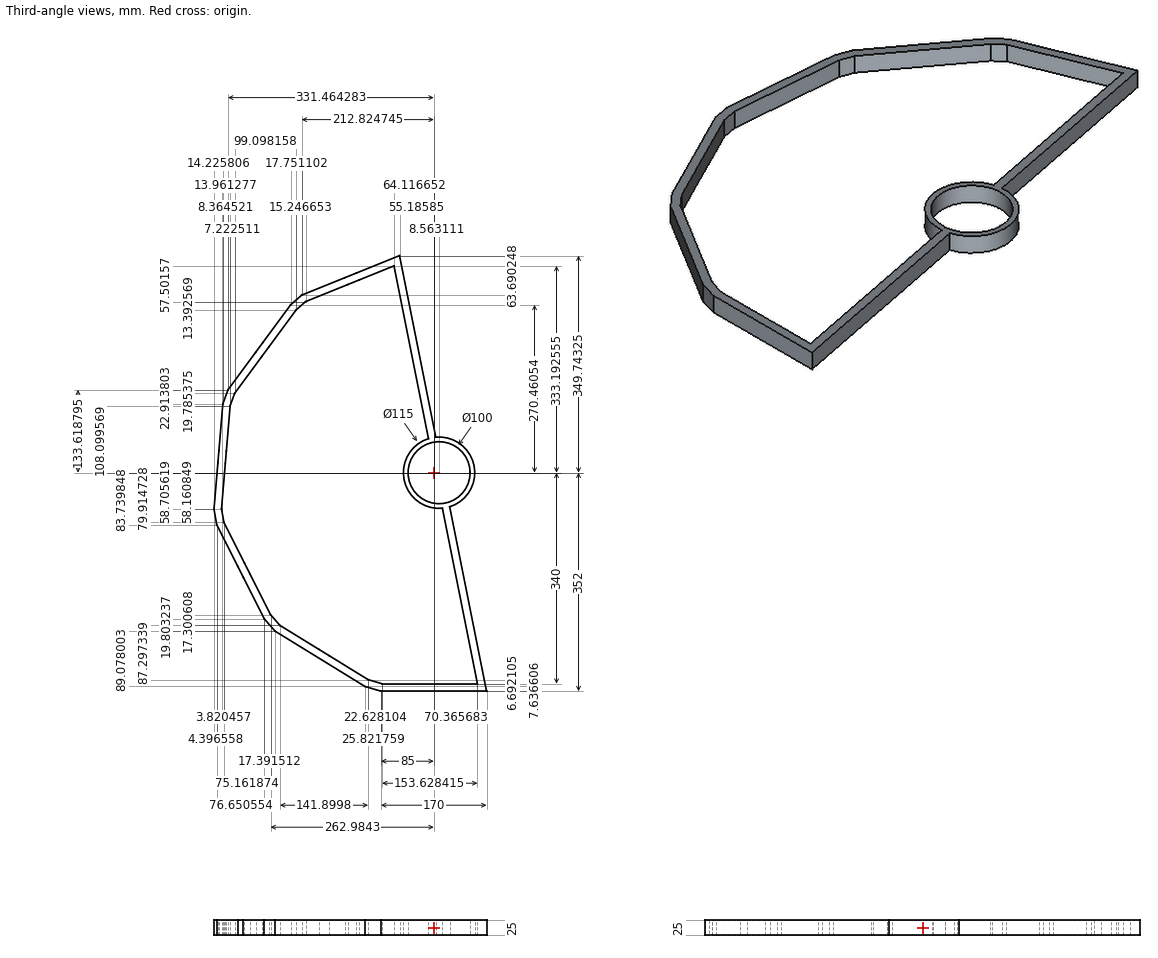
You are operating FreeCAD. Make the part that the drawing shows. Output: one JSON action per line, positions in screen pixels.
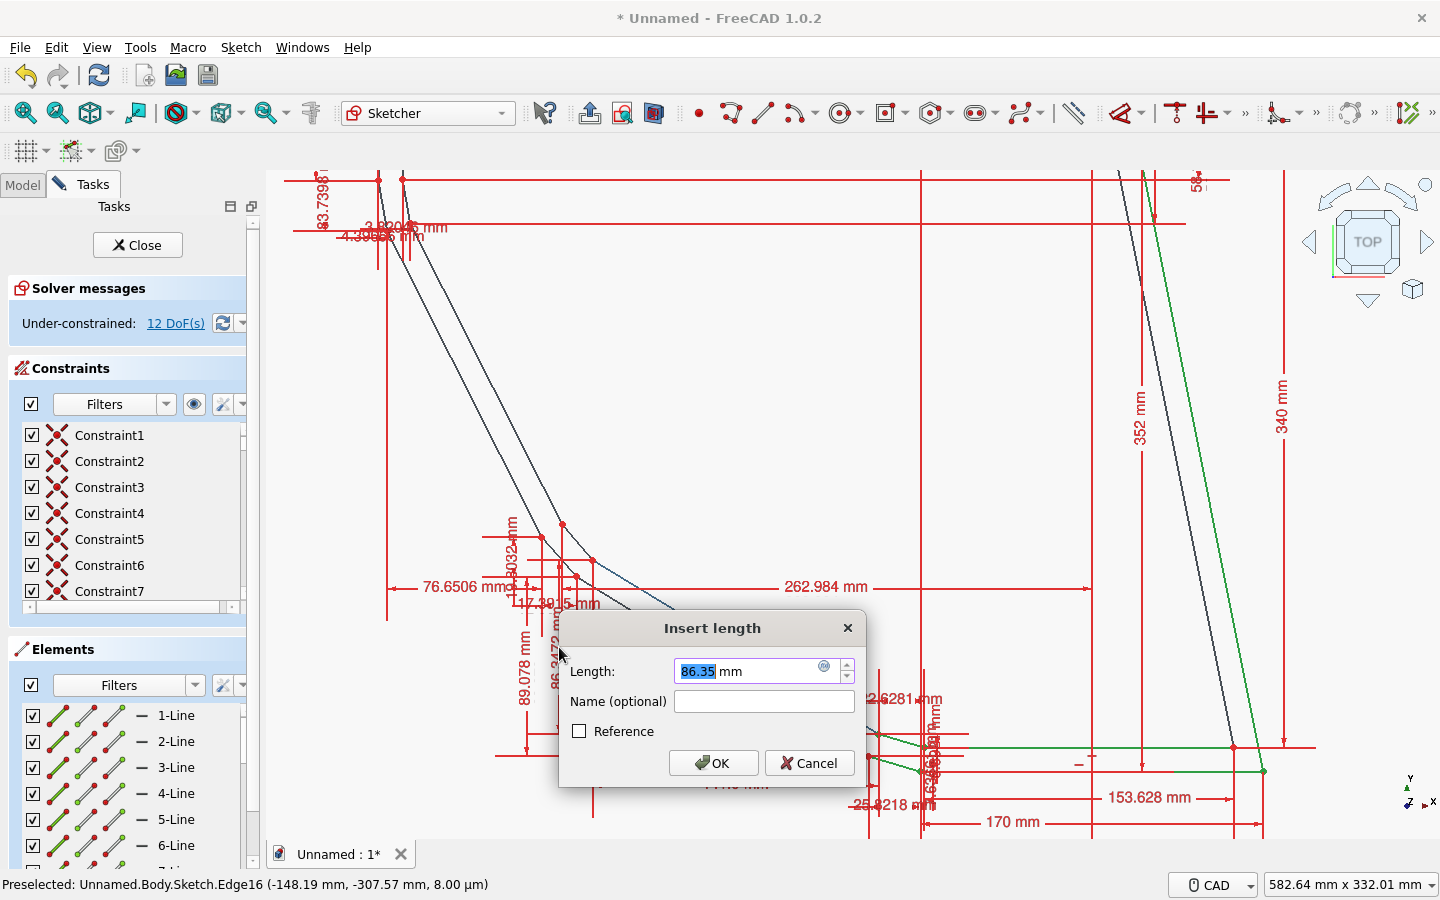
{"action": "type", "text": "87.297339"}
{"action": "key", "text": "Return"}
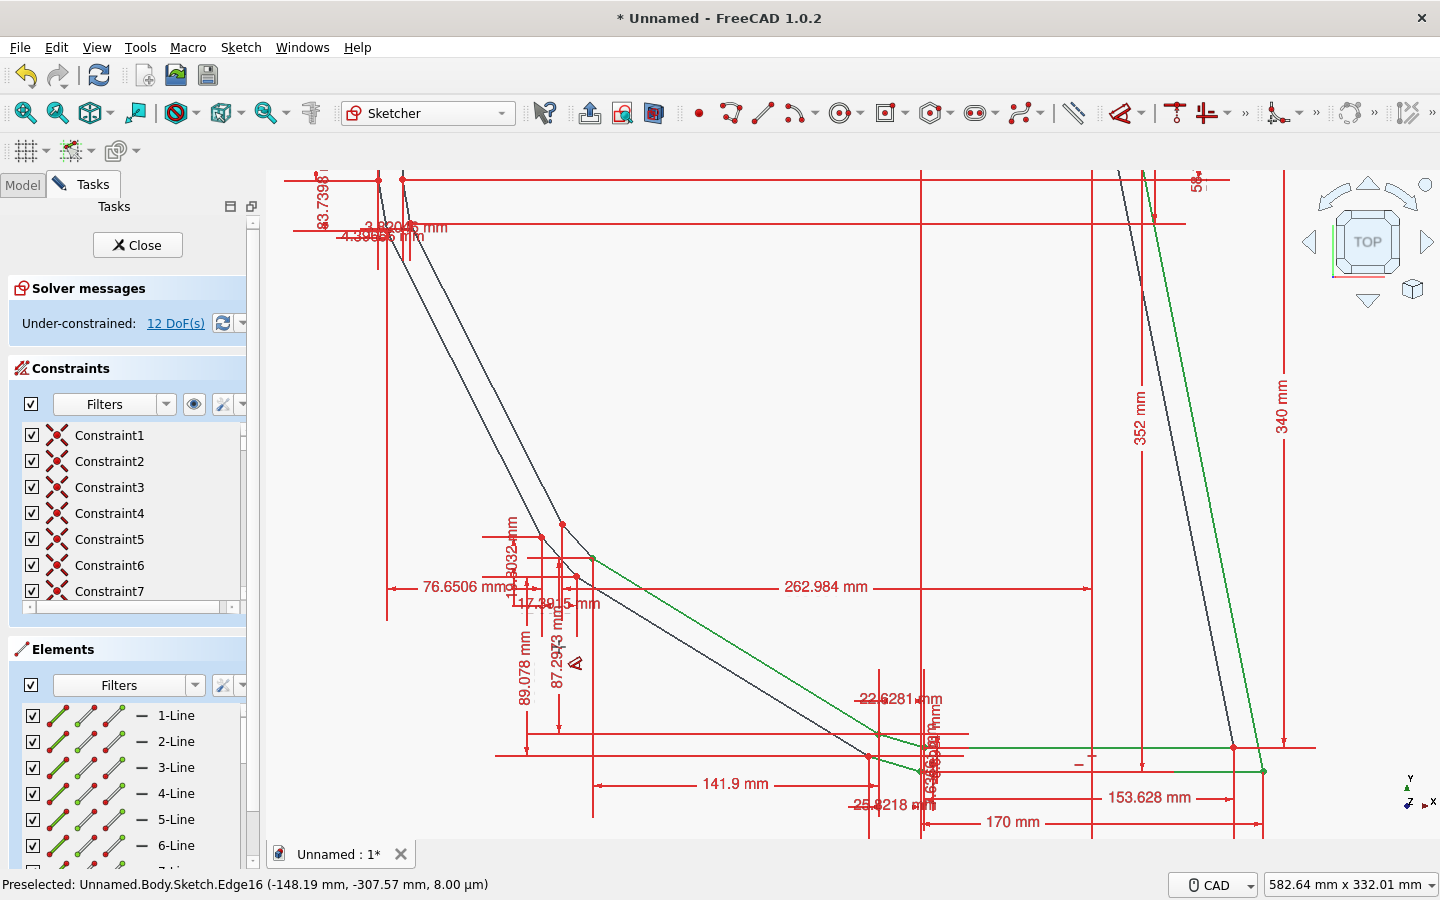
{"action": "left_click", "coordinate": [584, 548]}
{"action": "left_click", "coordinate": [627, 541]}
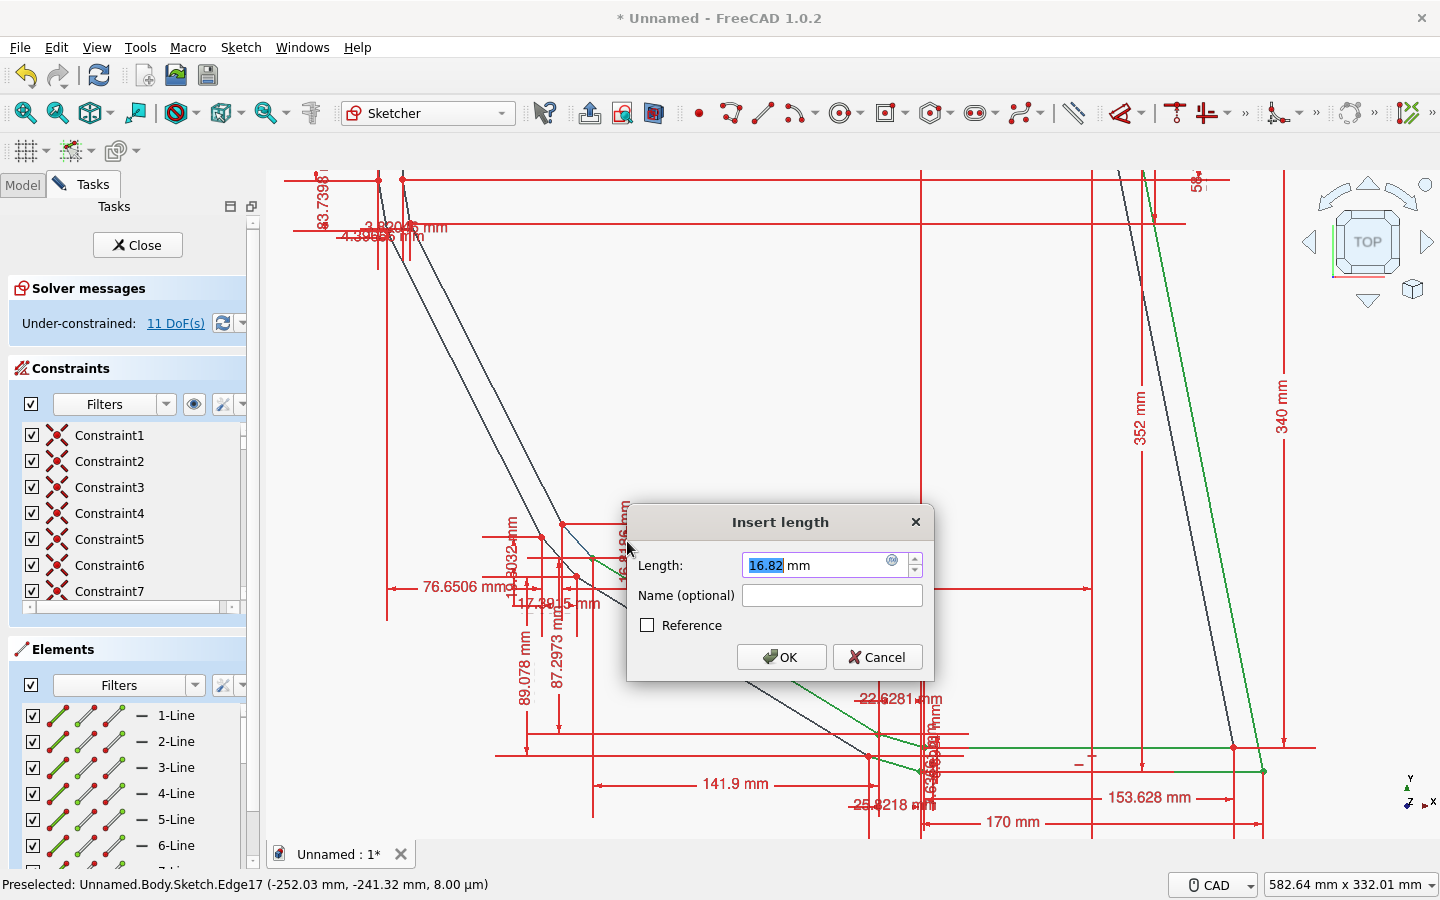
{"action": "type", "text": "17.300608"}
{"action": "key", "text": "Return"}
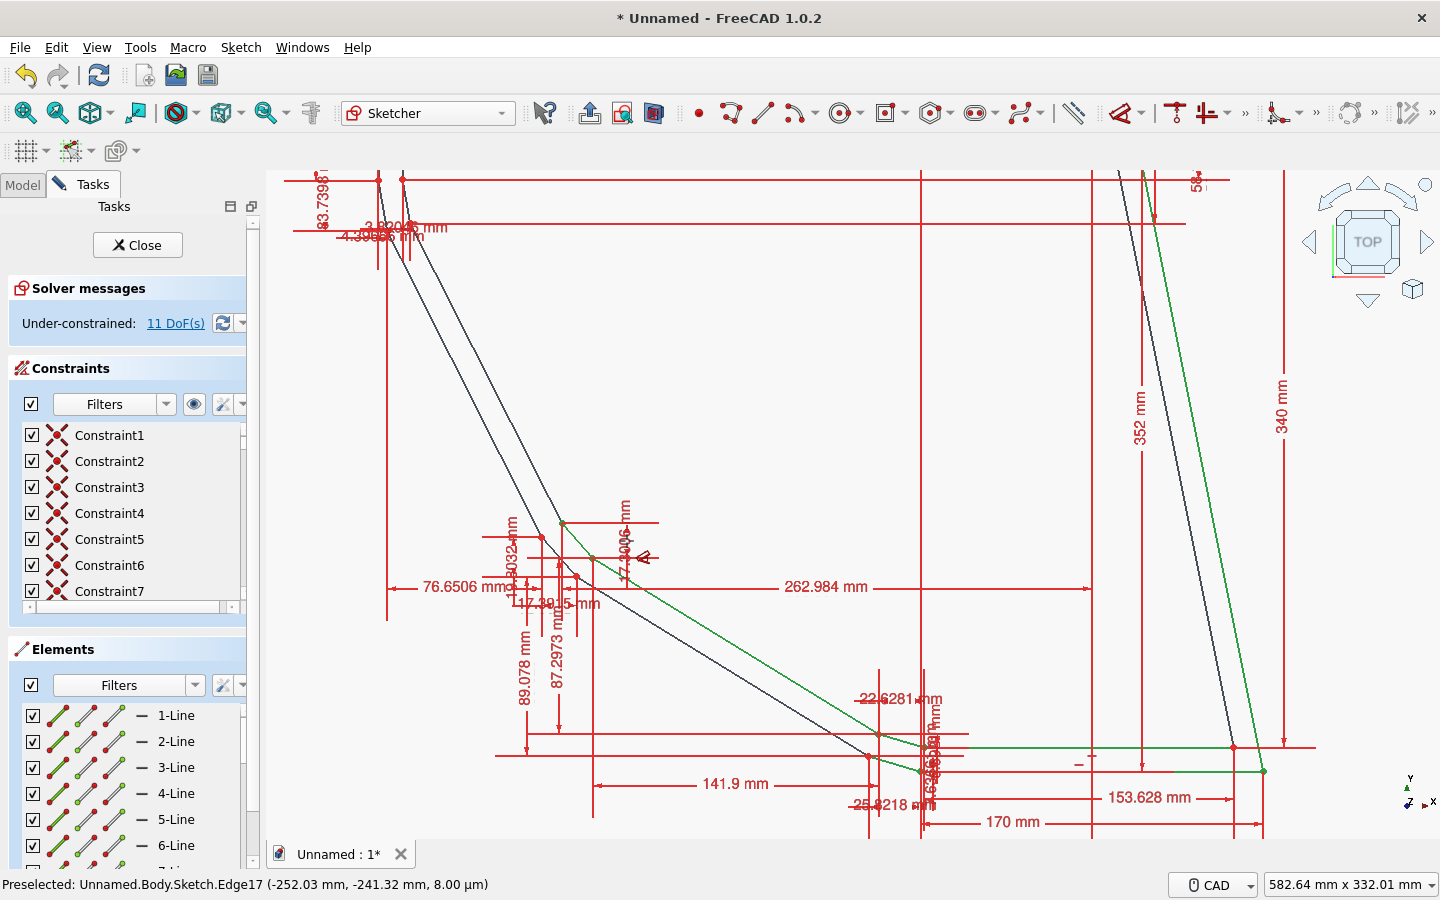
{"action": "left_click", "coordinate": [517, 433]}
{"action": "left_click", "coordinate": [433, 557]}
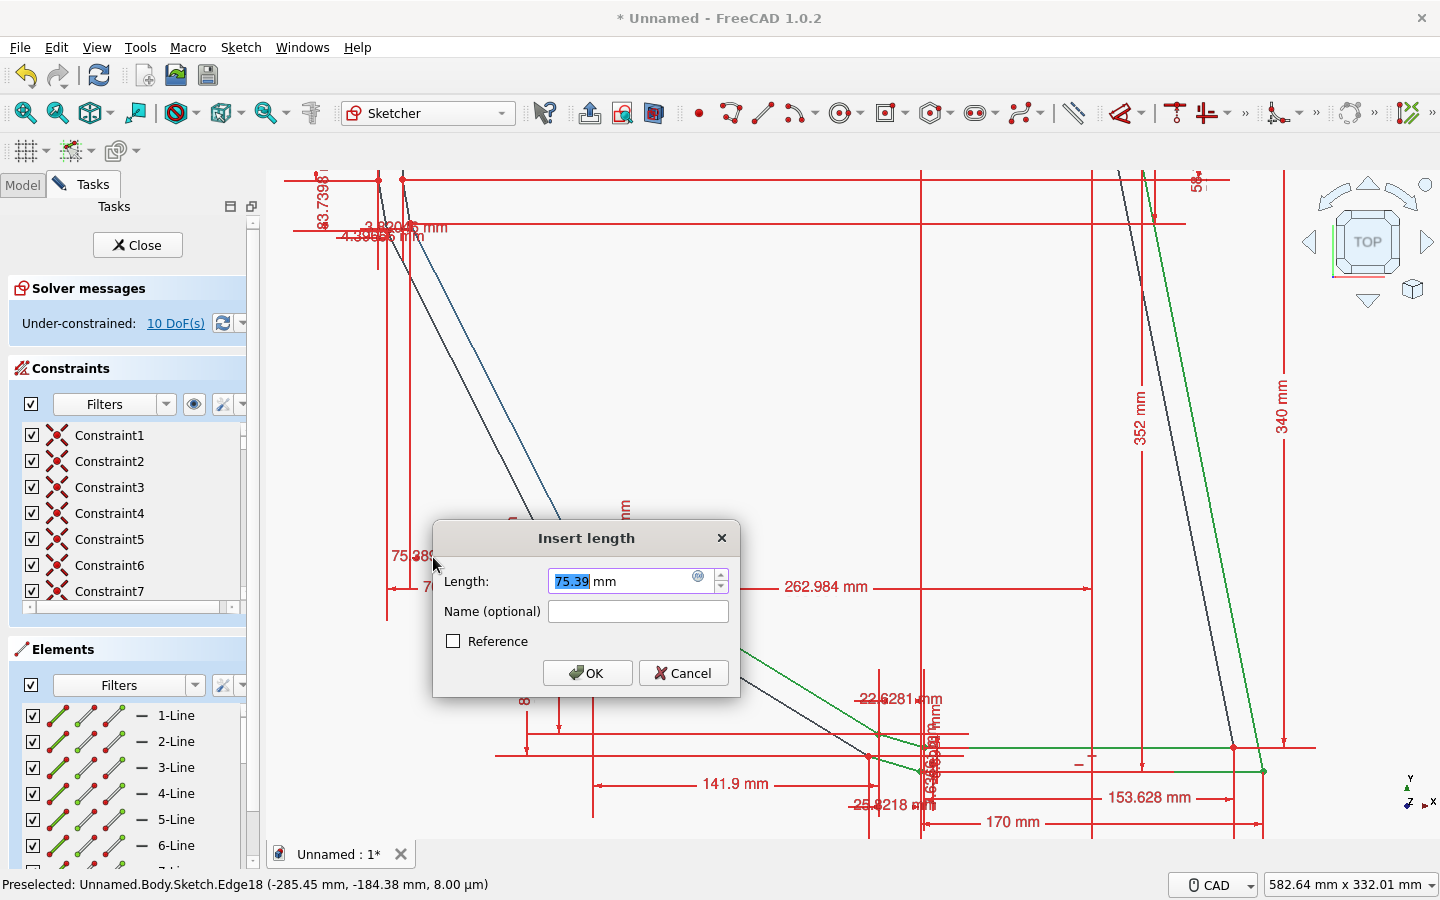
{"action": "type", "text": "75.161874"}
{"action": "key", "text": "Return"}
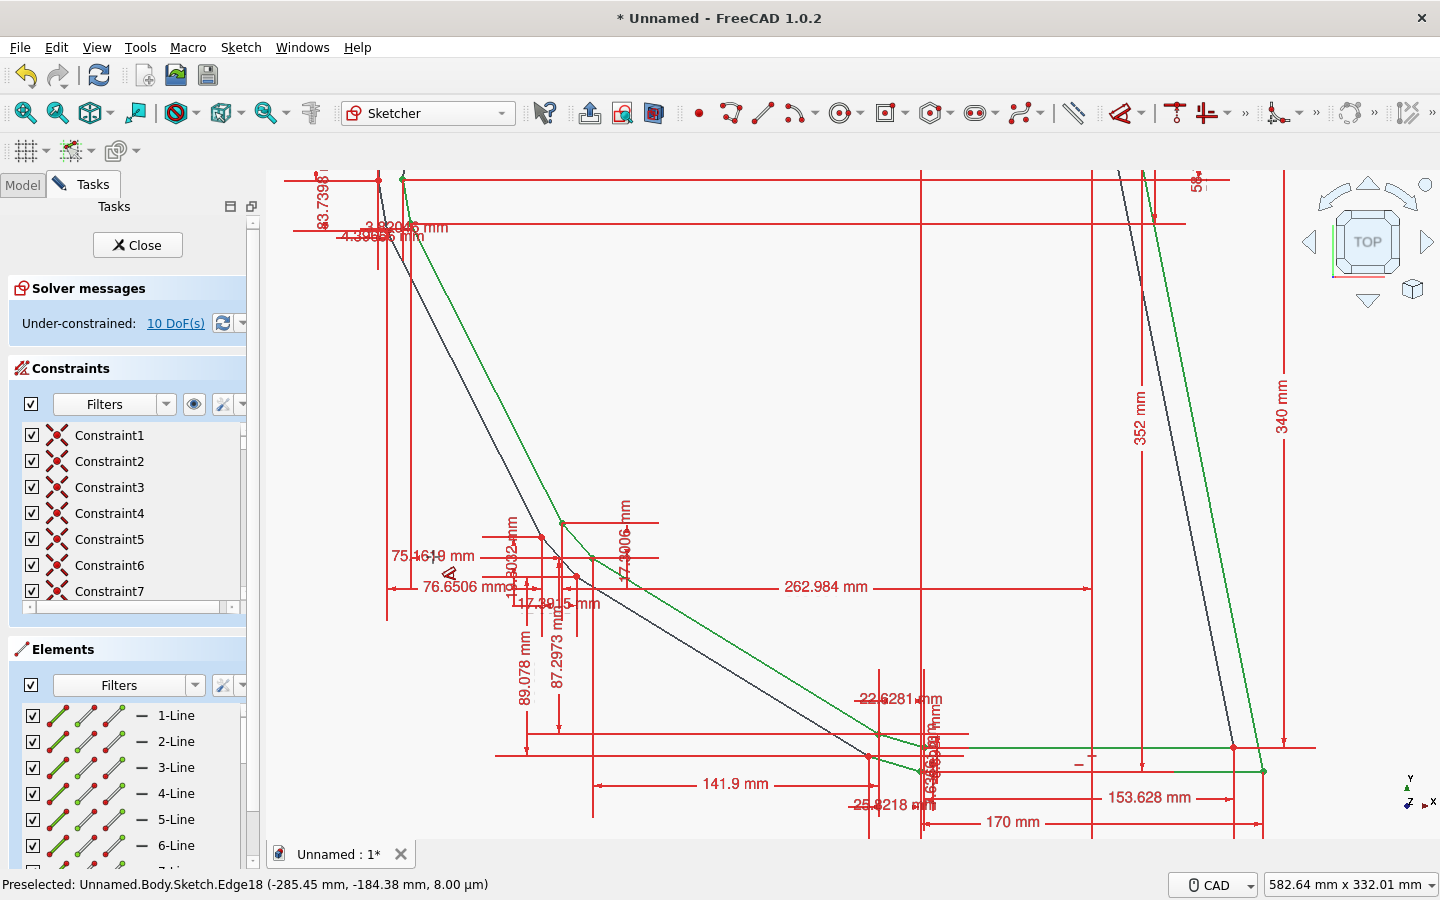
{"action": "scroll", "coordinate": [769, 694], "scroll_direction": "down", "scroll_amount": 6}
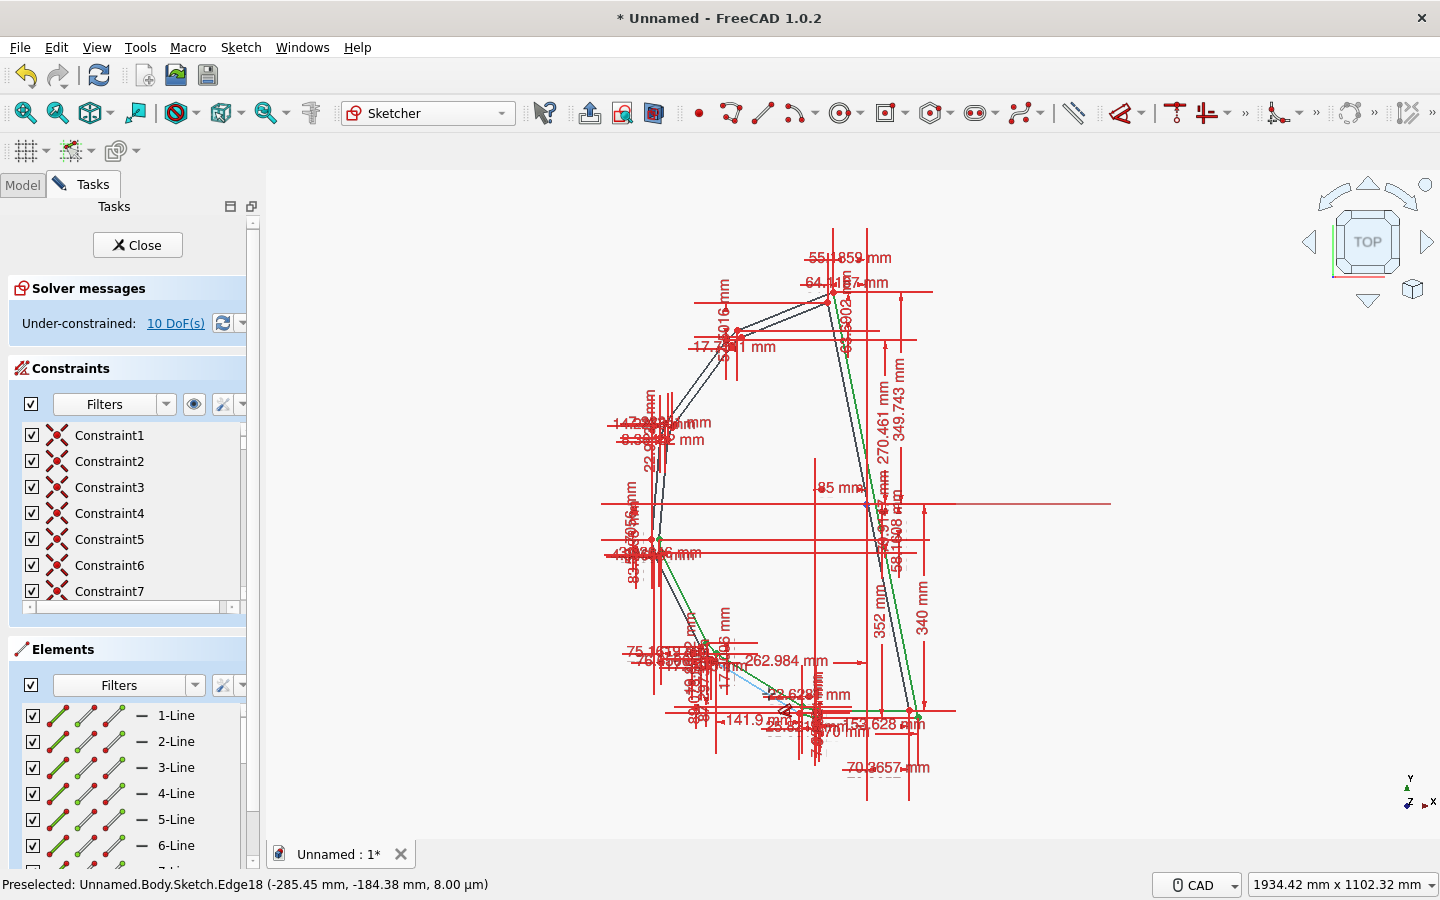
{"action": "scroll", "coordinate": [662, 509], "scroll_direction": "up", "scroll_amount": 8}